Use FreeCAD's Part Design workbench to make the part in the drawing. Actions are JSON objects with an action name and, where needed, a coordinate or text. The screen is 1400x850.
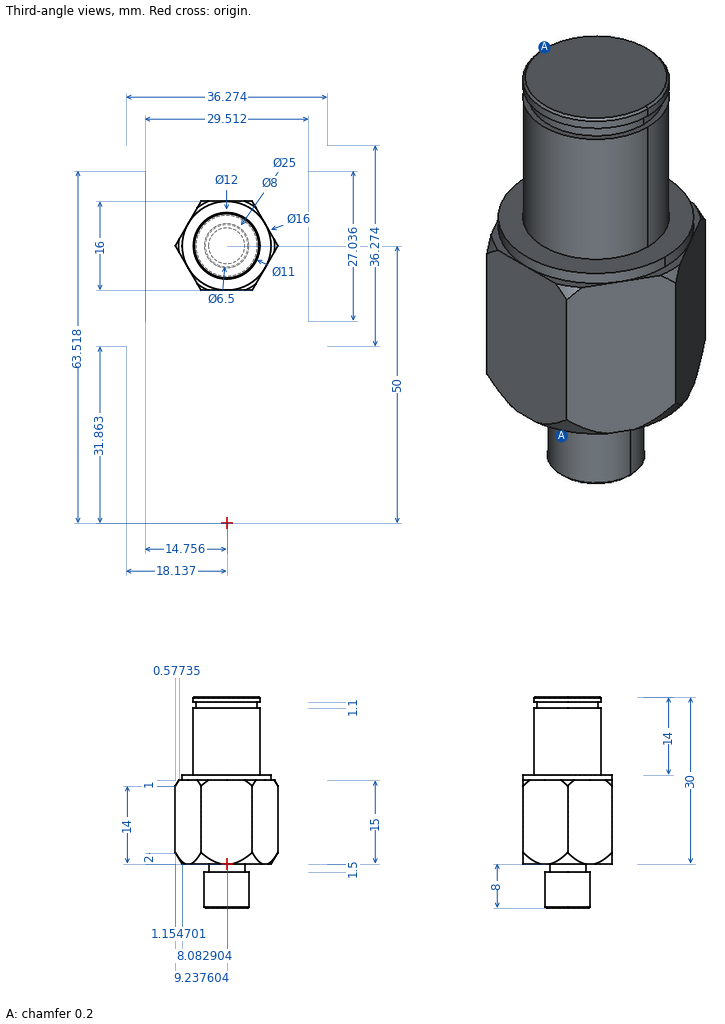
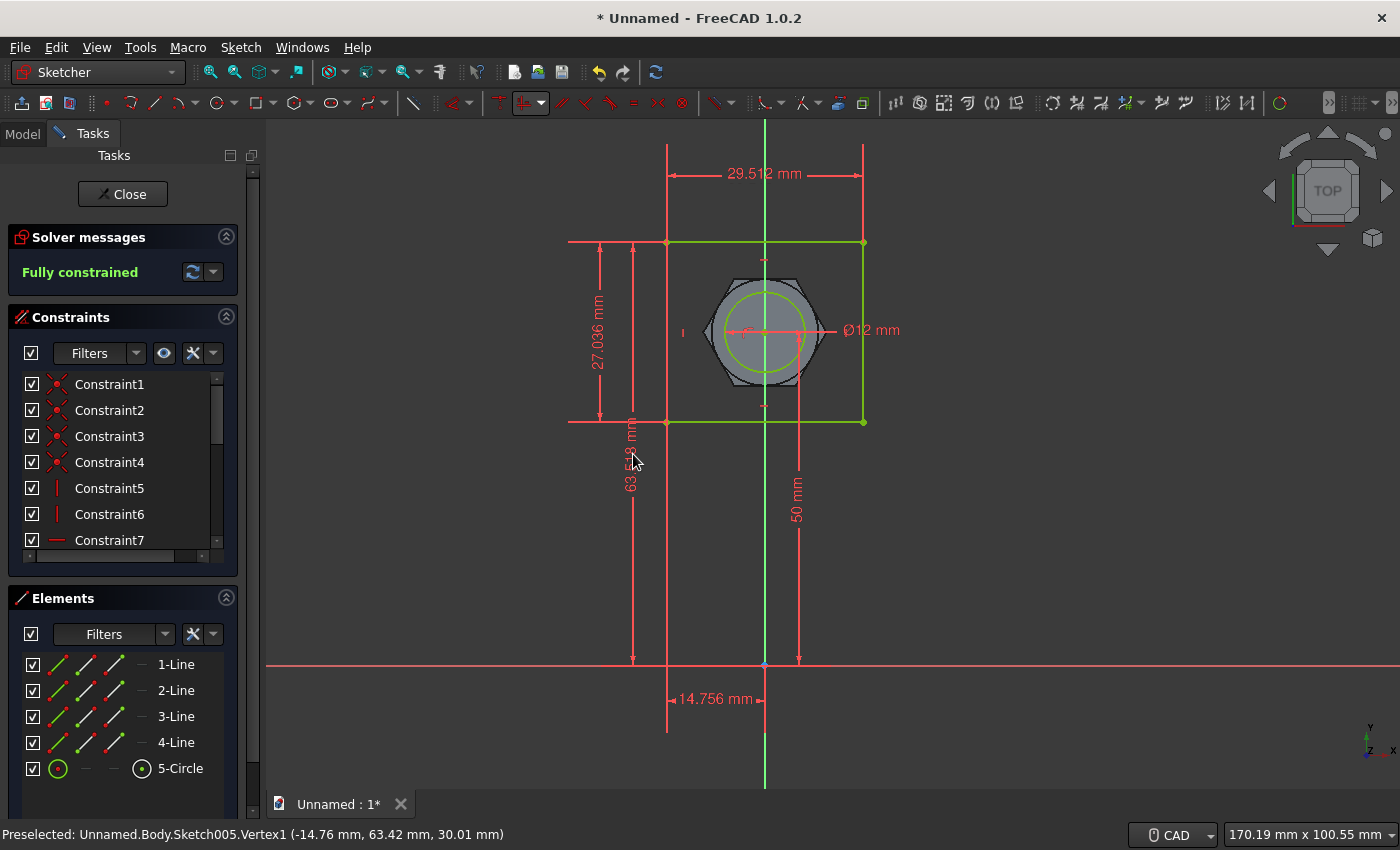
{"action": "left_click", "coordinate": [123, 194]}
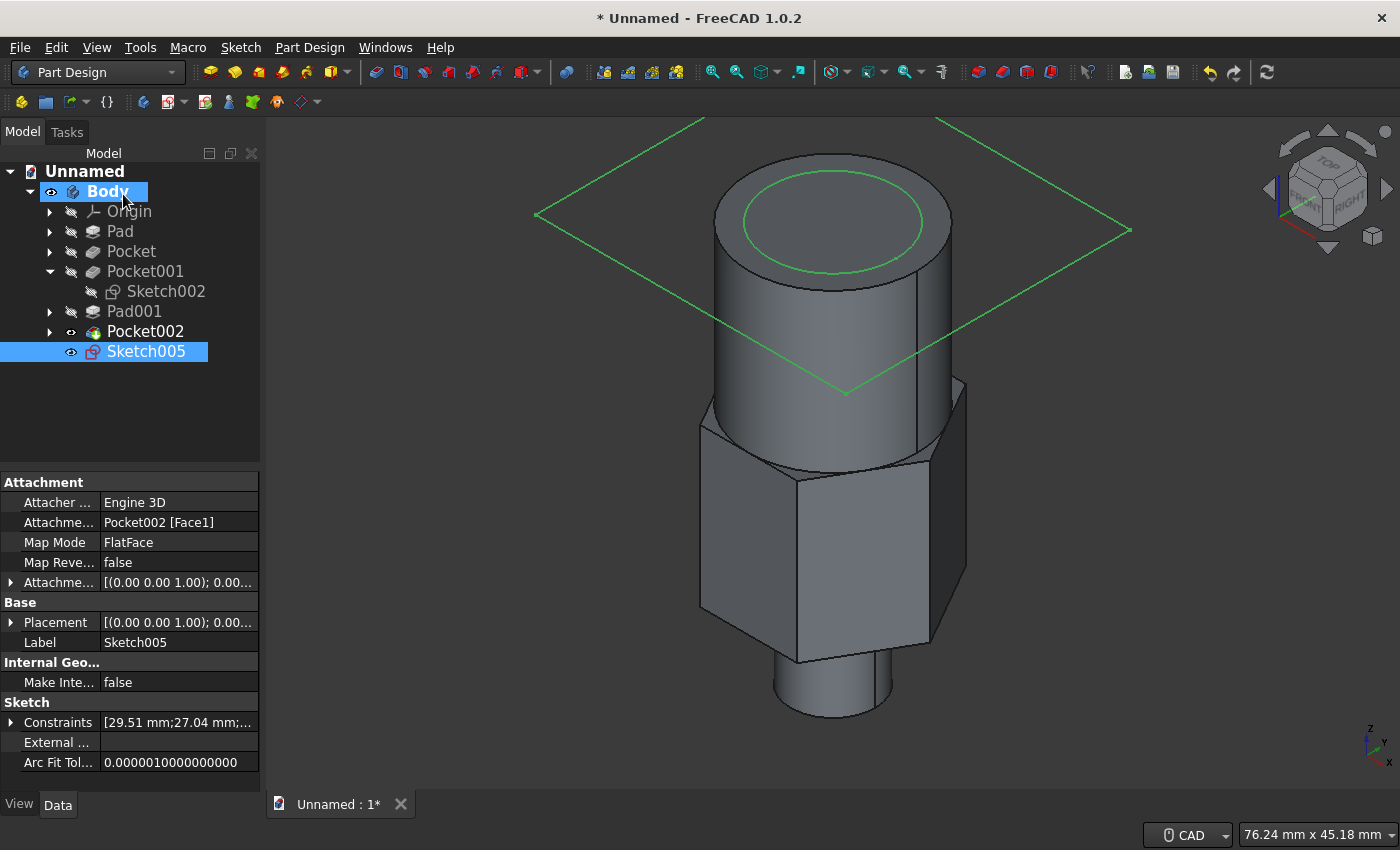
{"action": "left_click", "coordinate": [378, 72]}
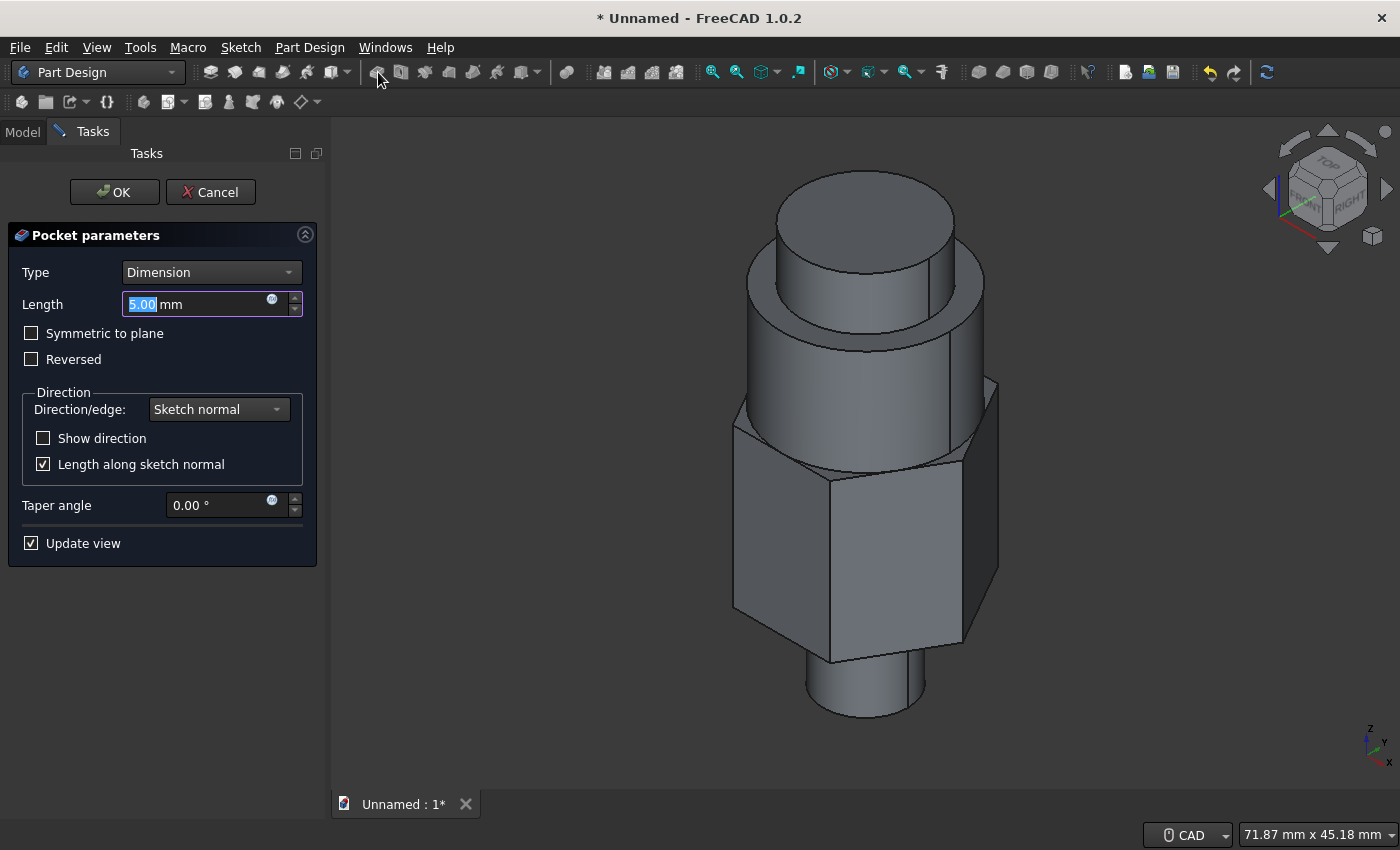
{"action": "type", "text": "14"}
{"action": "key", "text": "Tab"}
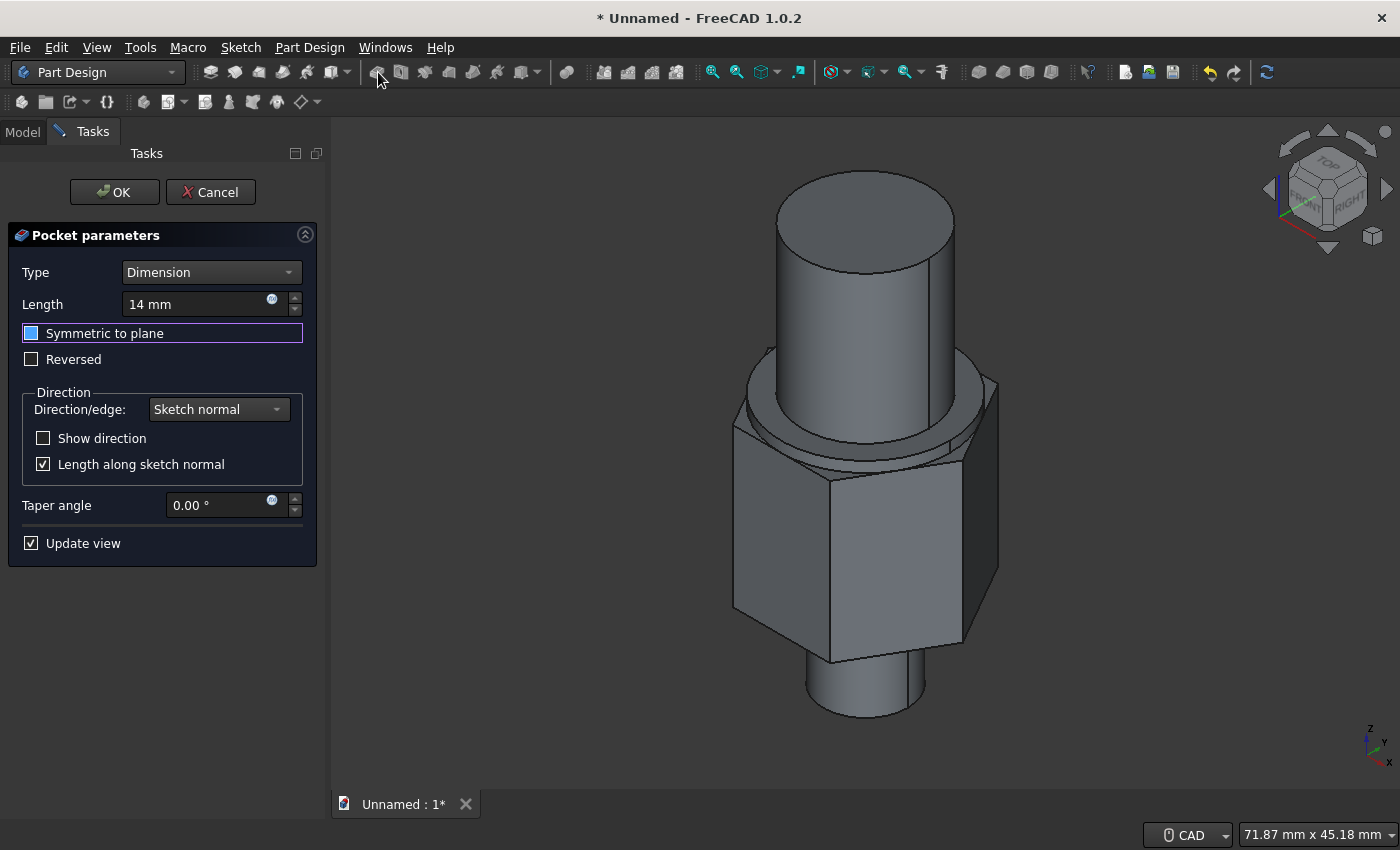
{"action": "left_click", "coordinate": [115, 192]}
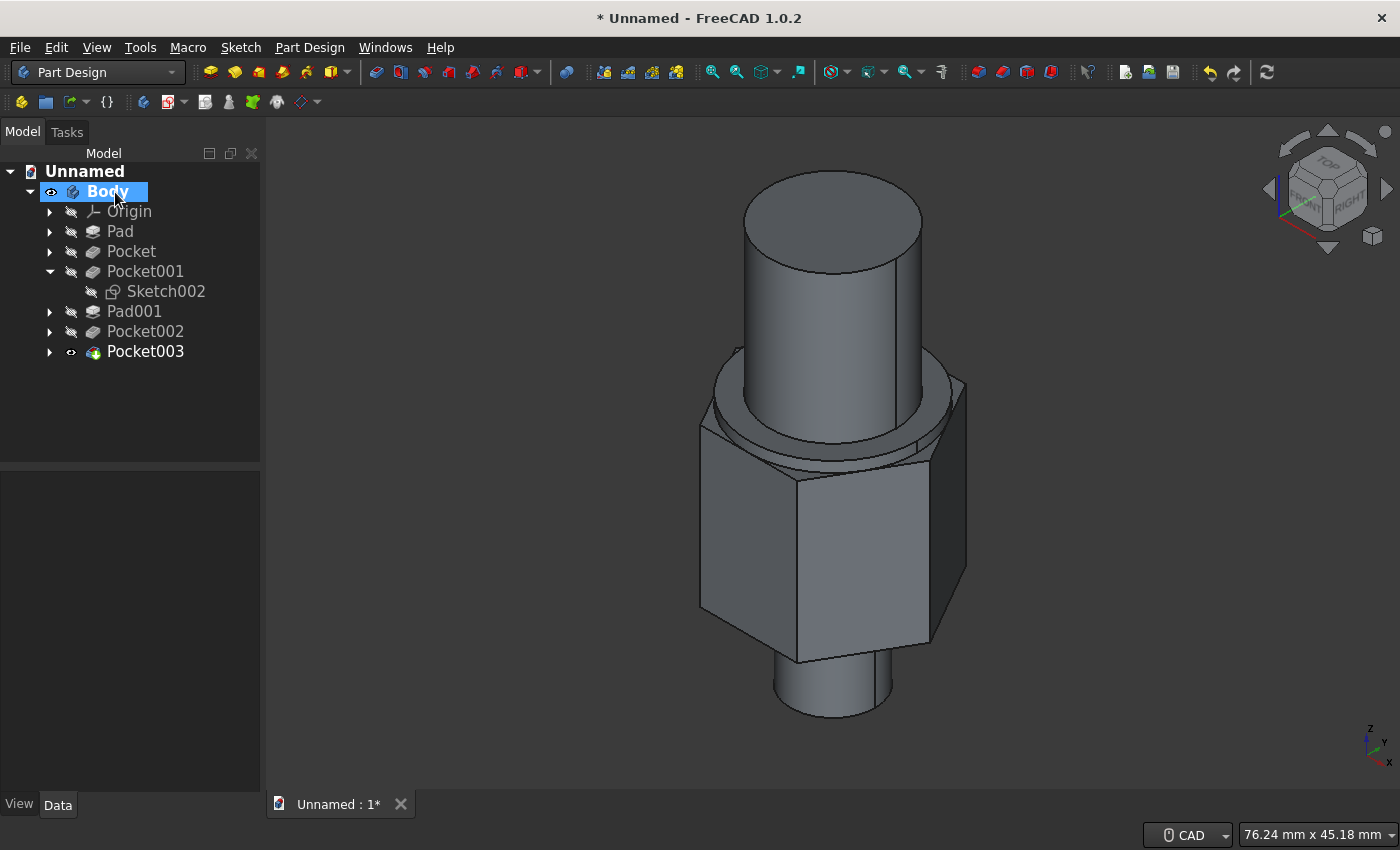
{"action": "left_click", "coordinate": [50, 212]}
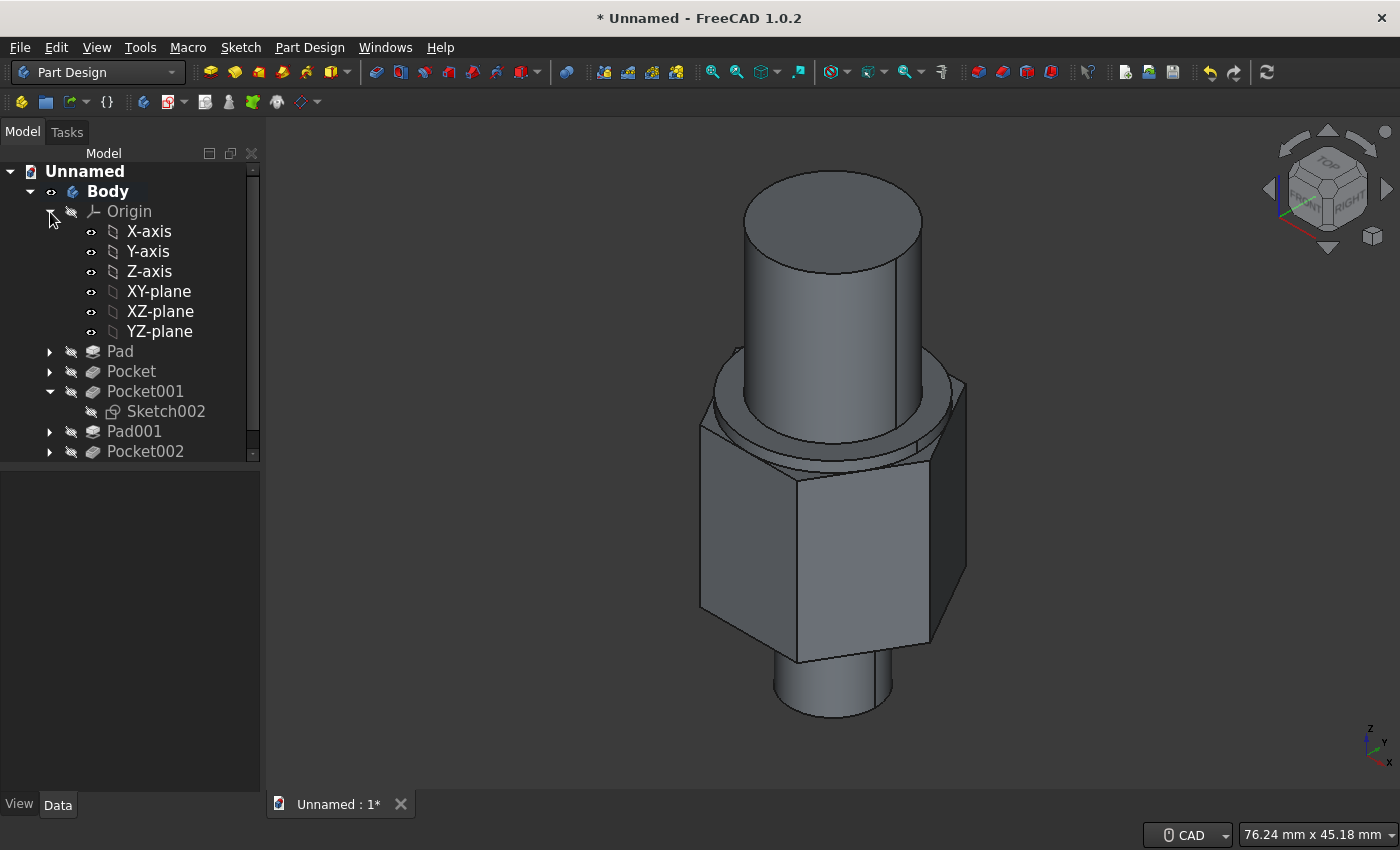
{"action": "left_click", "coordinate": [136, 292]}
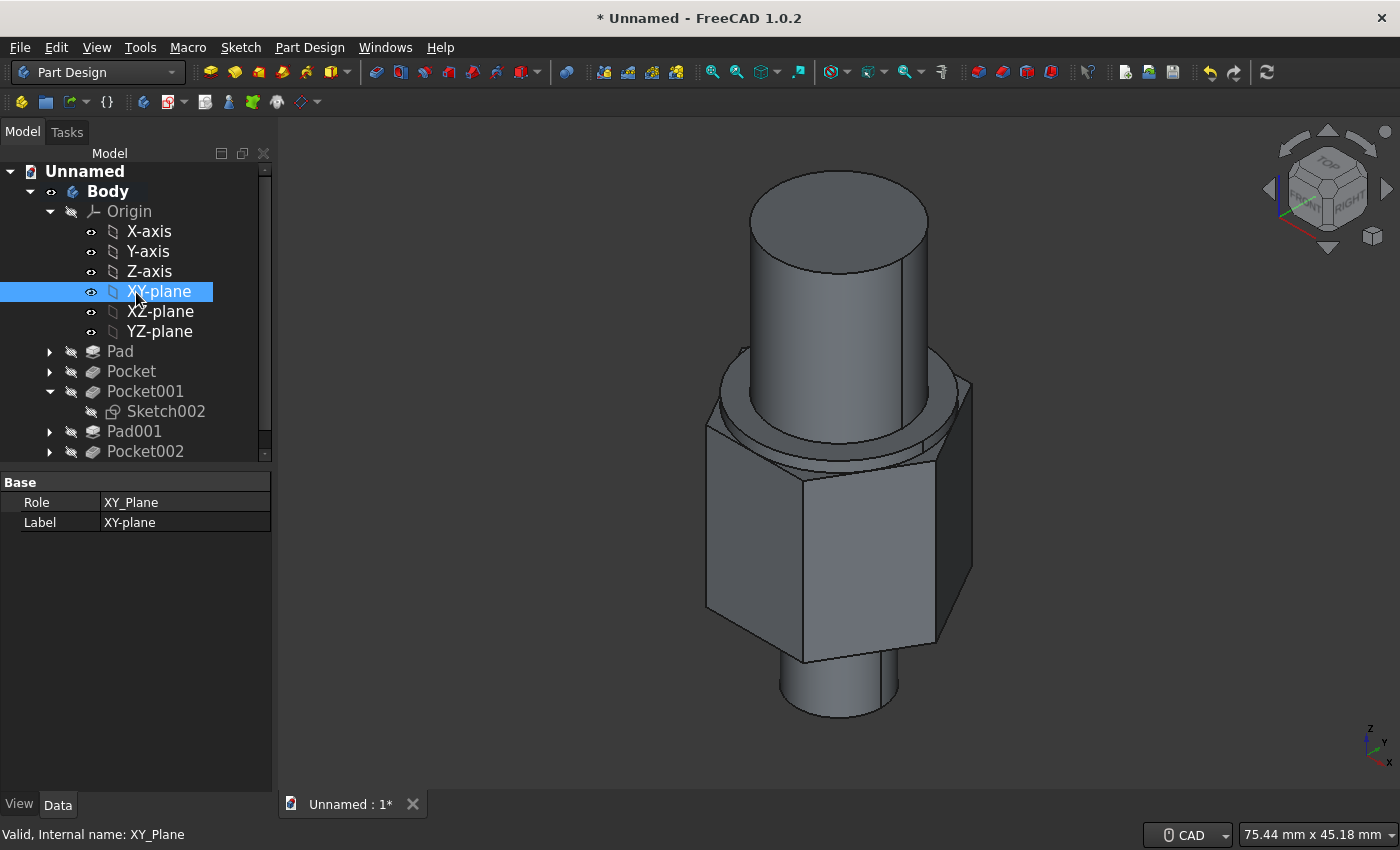
{"action": "left_click", "coordinate": [302, 102]}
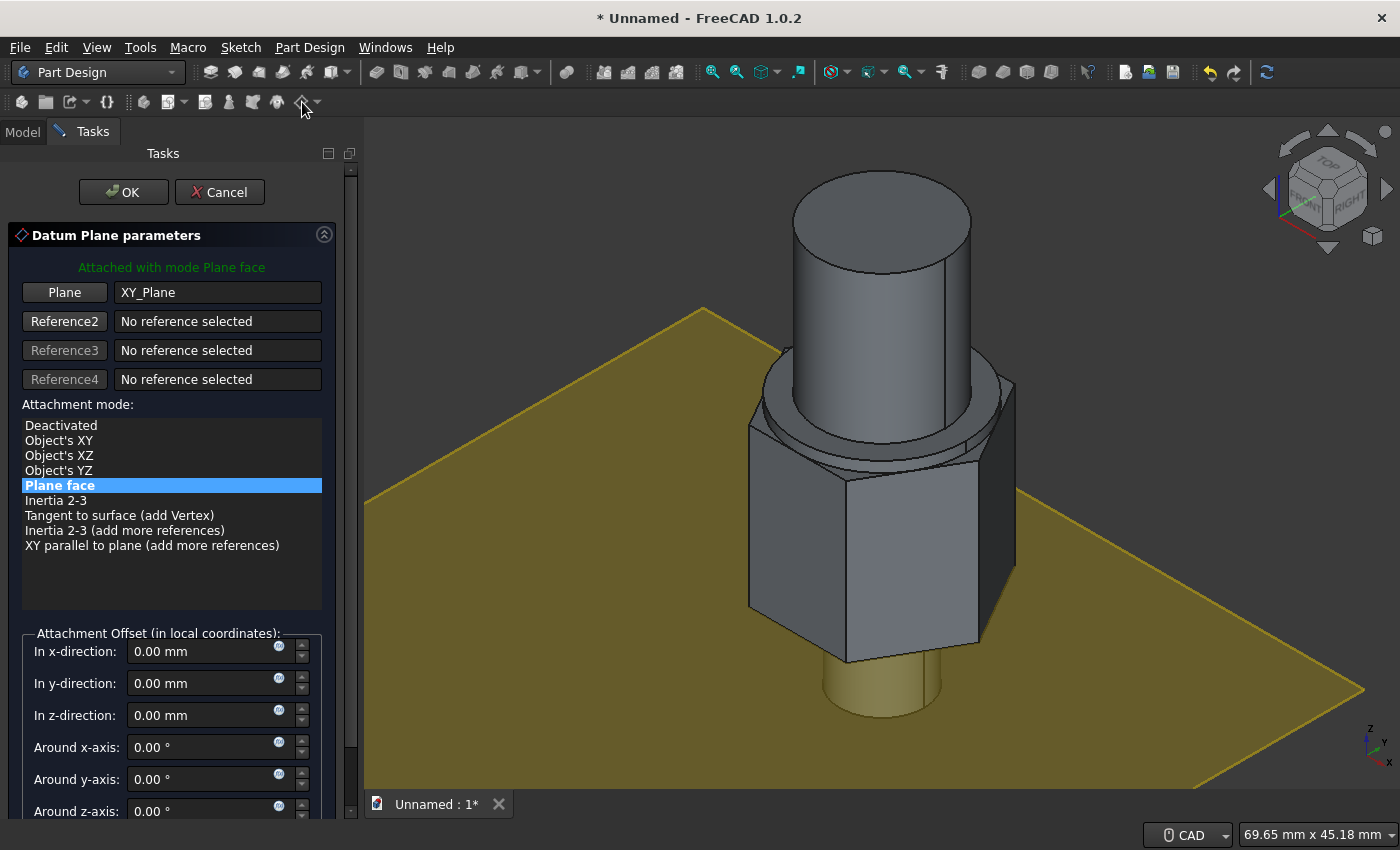
{"action": "triple_click", "coordinate": [210, 715]}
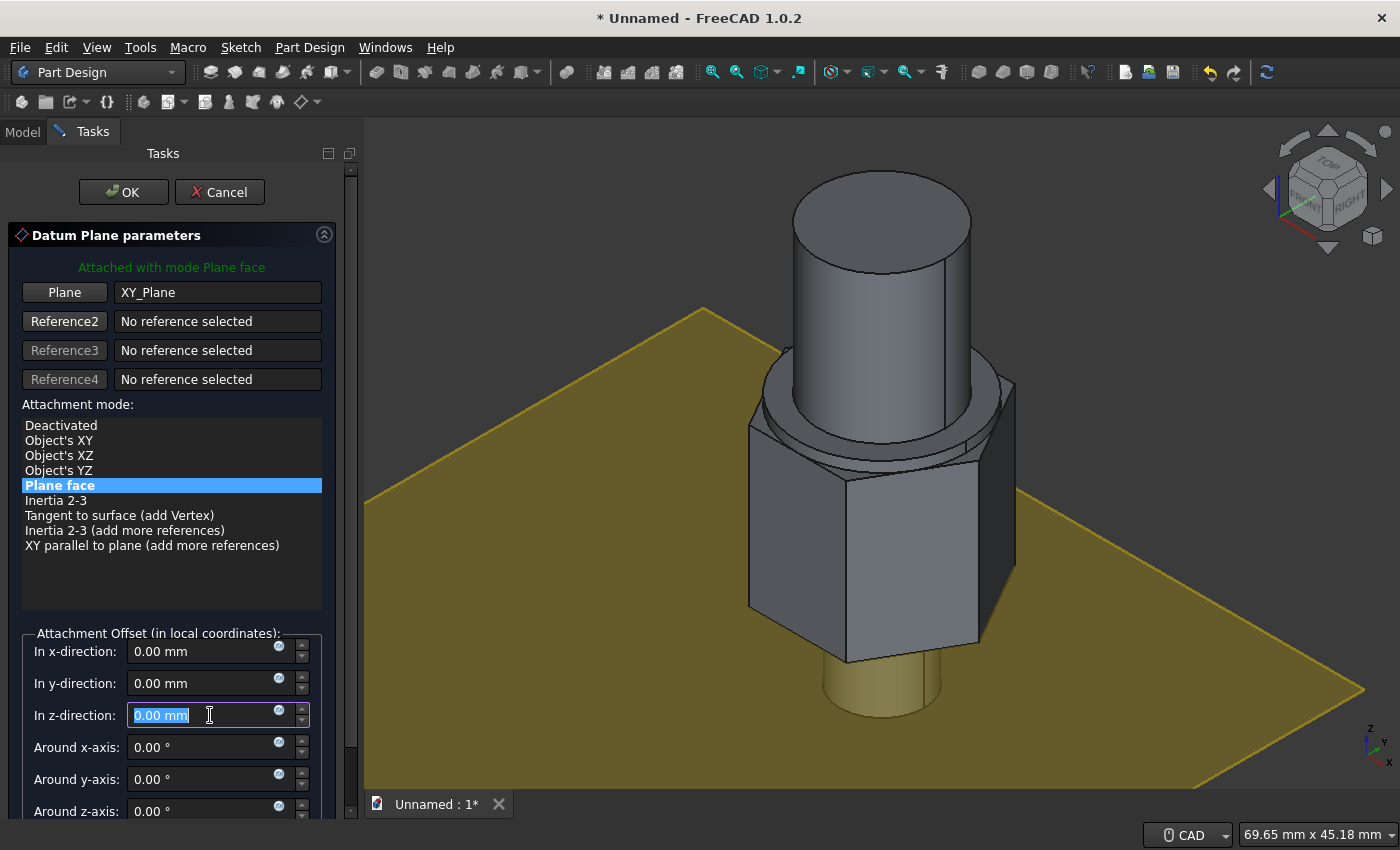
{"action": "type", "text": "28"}
{"action": "key", "text": "Tab"}